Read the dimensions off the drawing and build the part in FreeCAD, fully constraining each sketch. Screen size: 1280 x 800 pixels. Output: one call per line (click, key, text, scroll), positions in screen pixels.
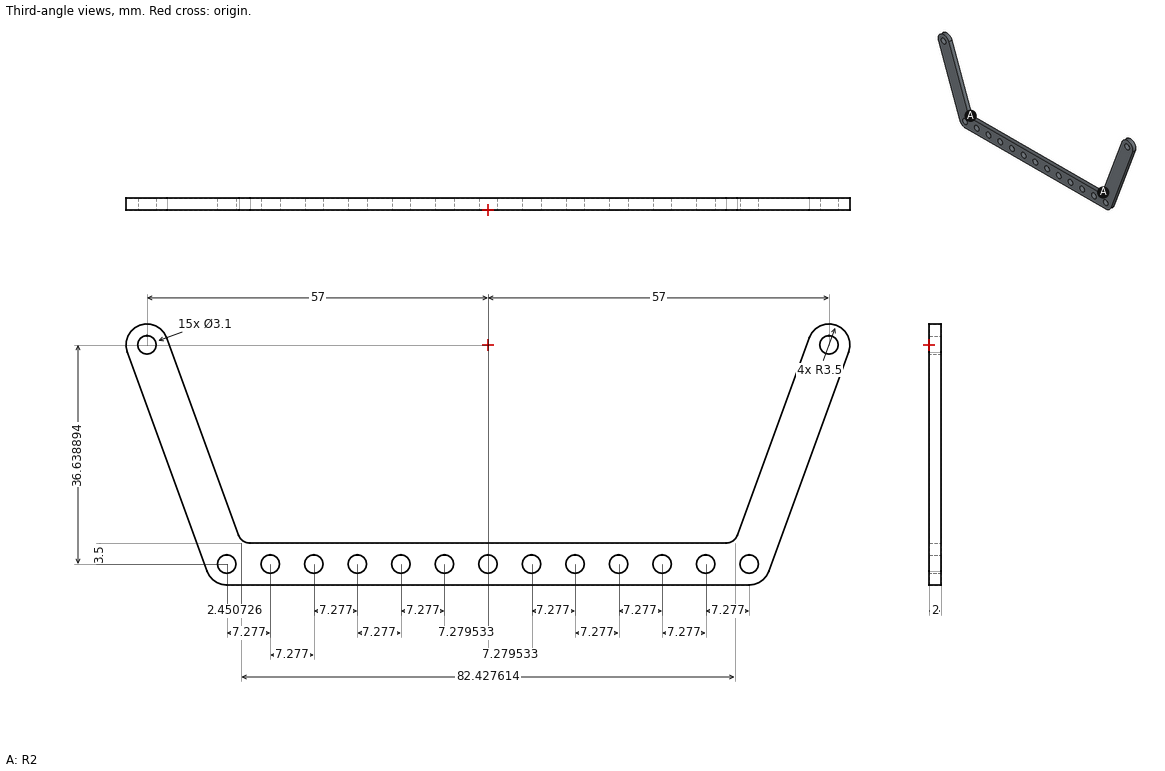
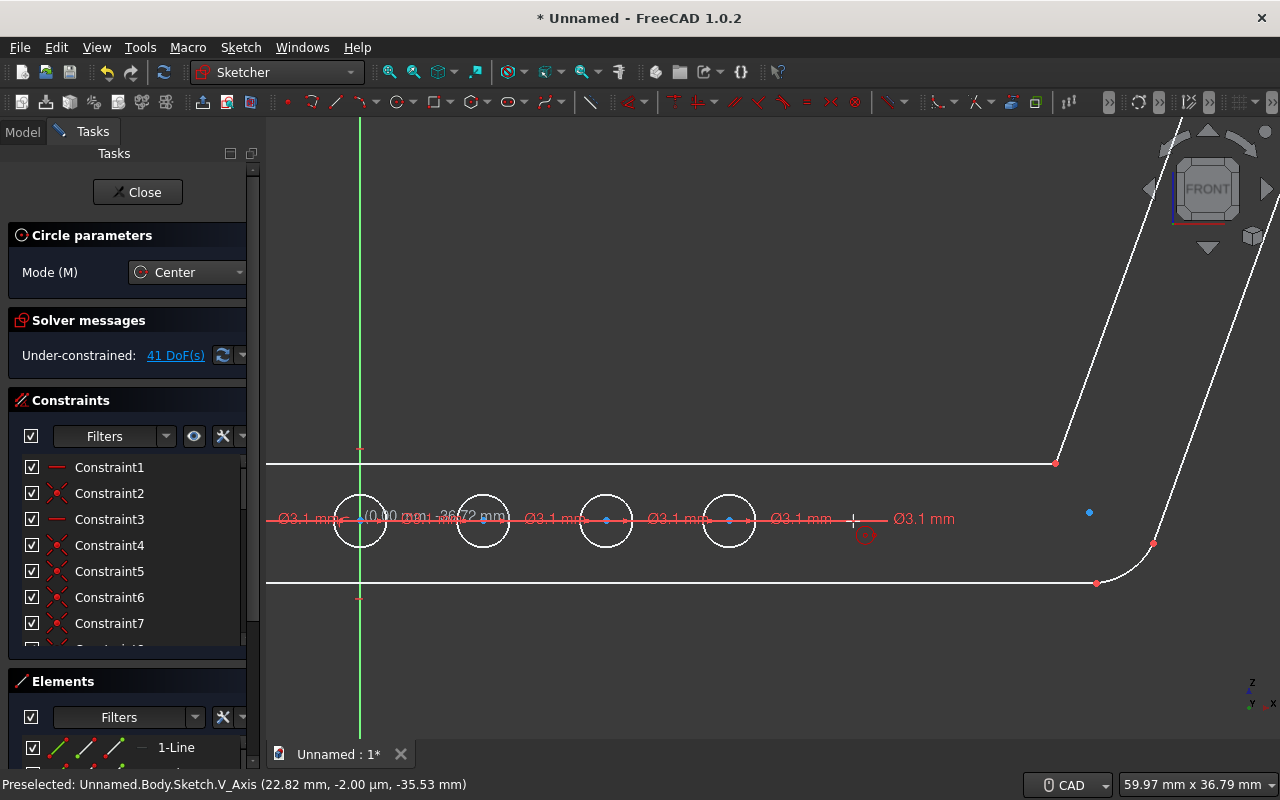
click(852, 520)
move(871, 501)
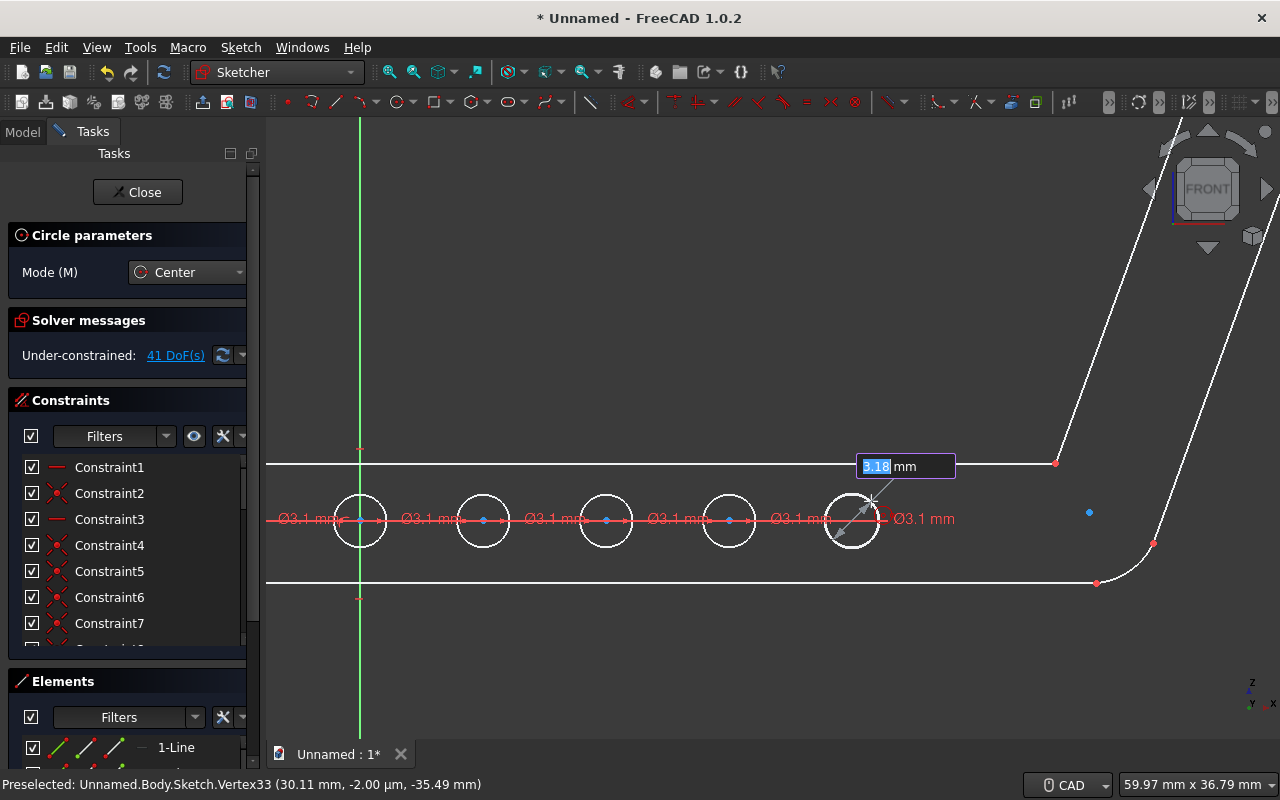
text(3.1)
key(Return)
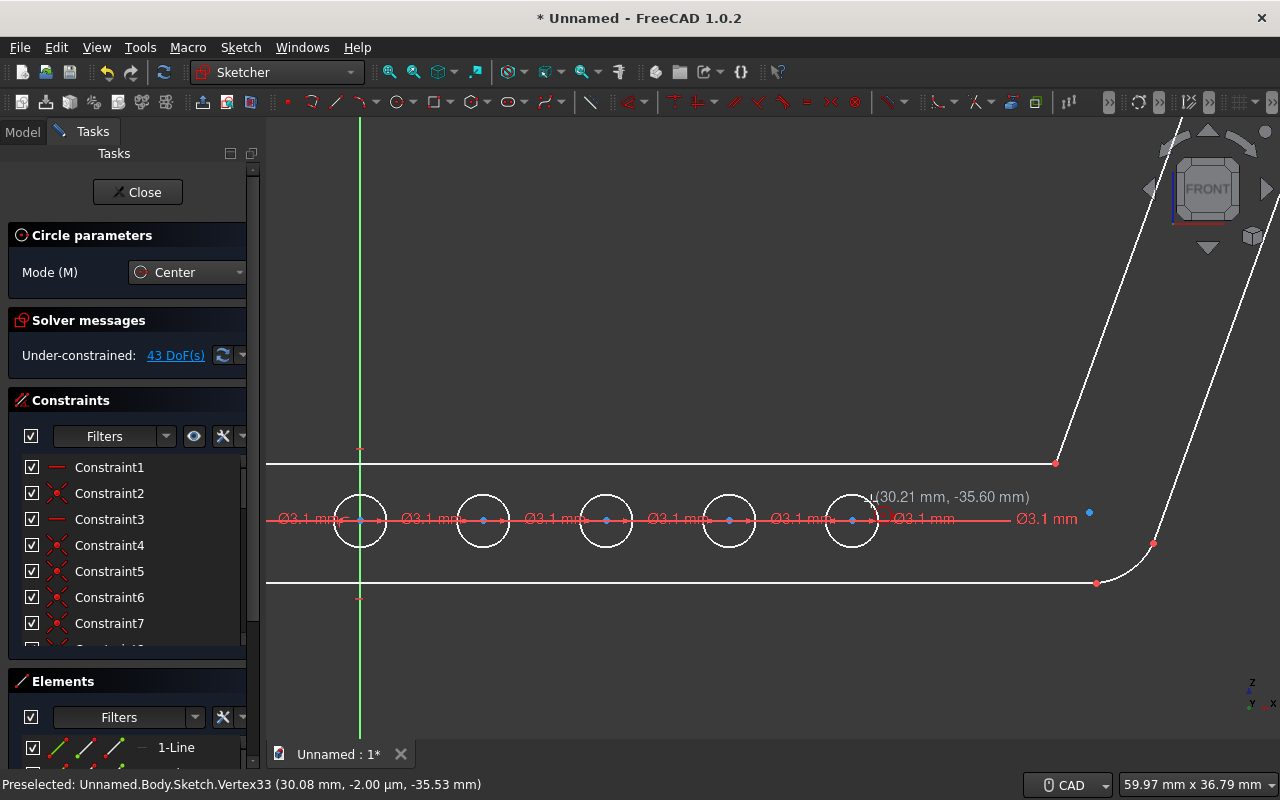
click(975, 520)
move(994, 501)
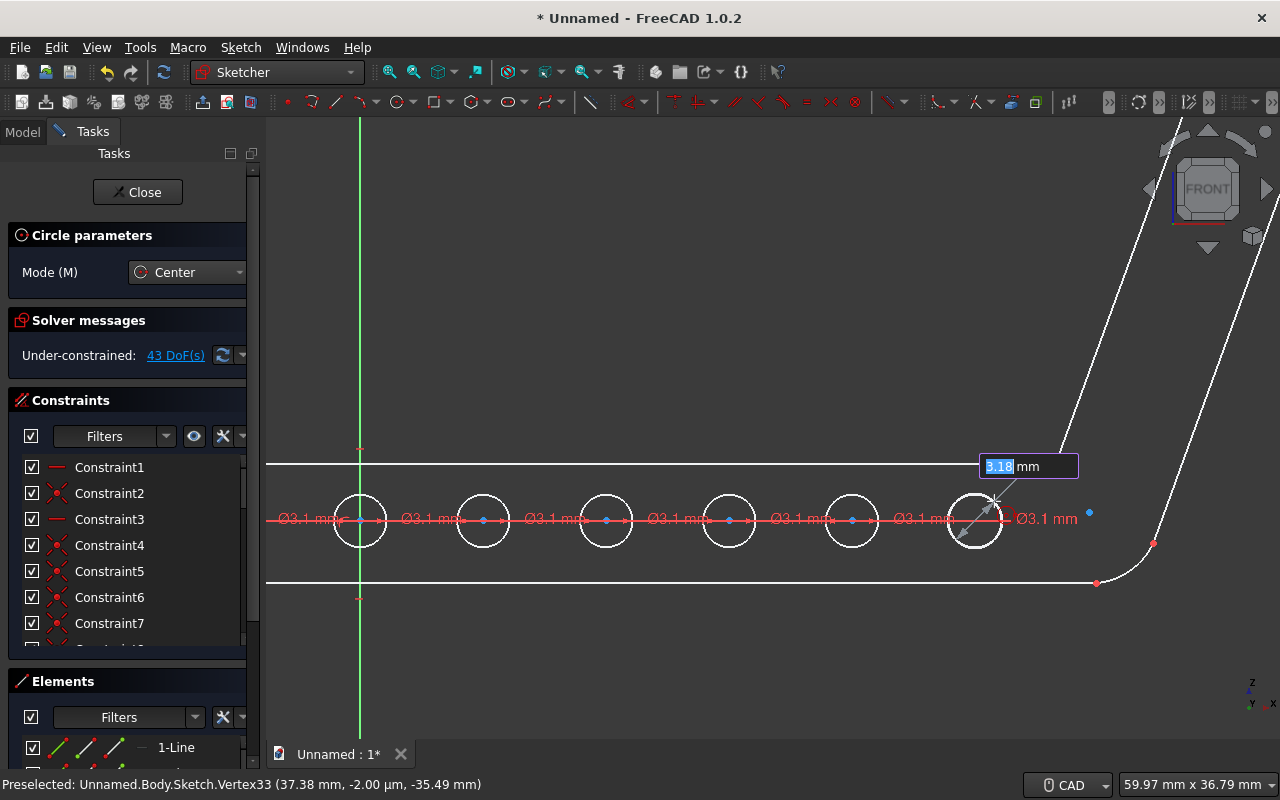
text(3.1)
key(Return)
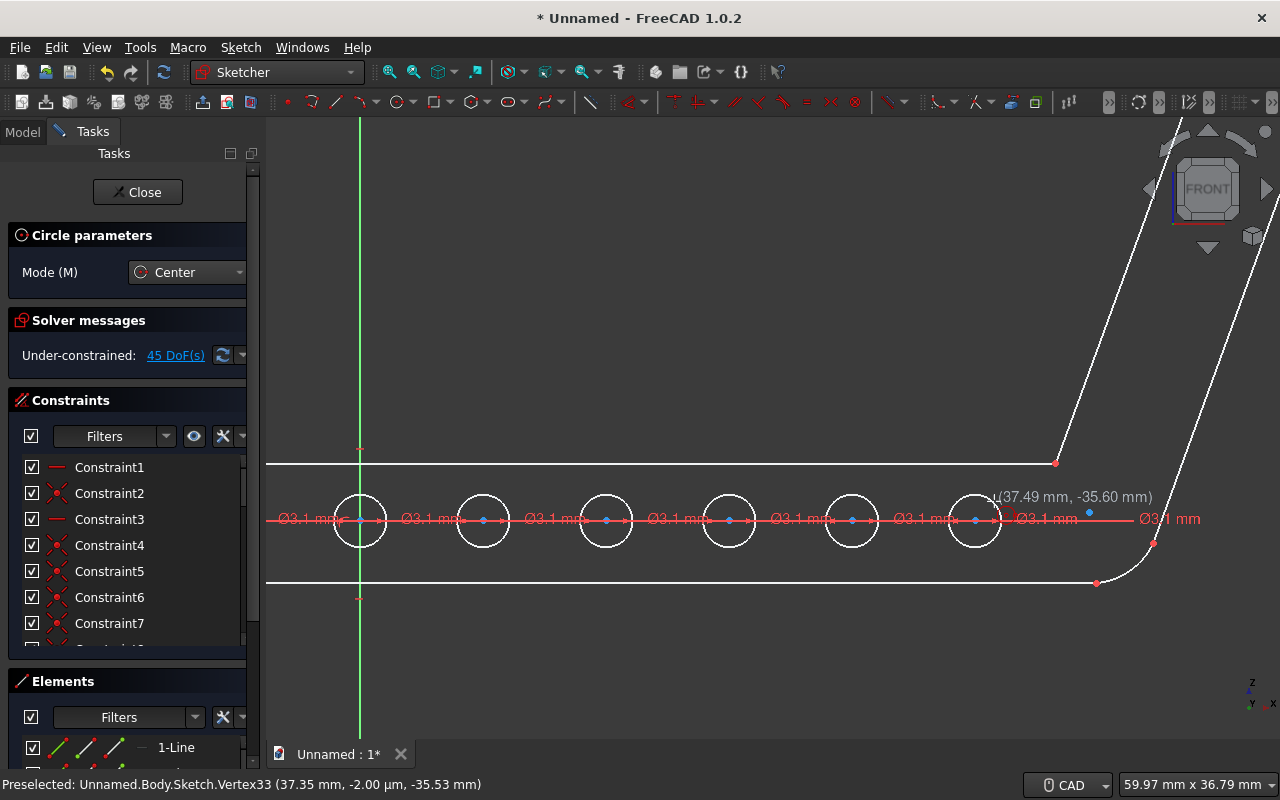
click(1098, 520)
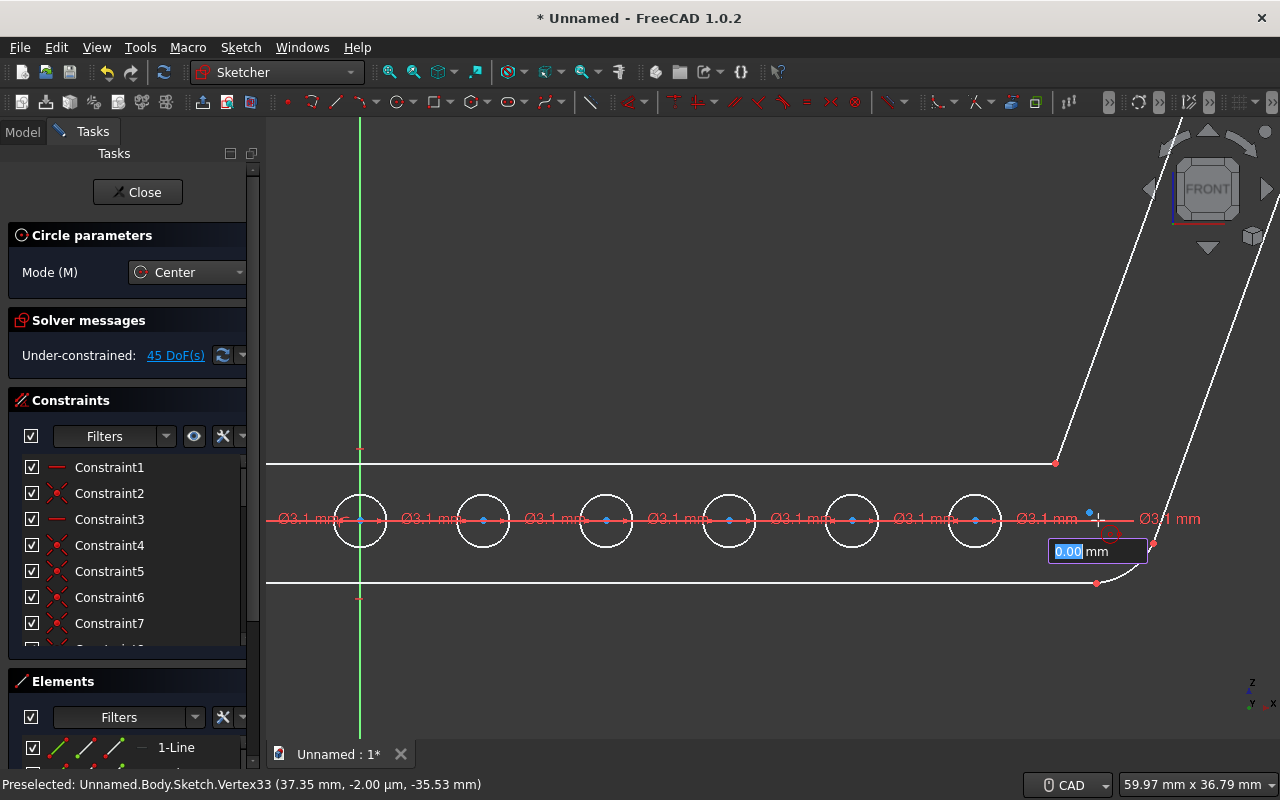
scroll(853, 521, down, 6)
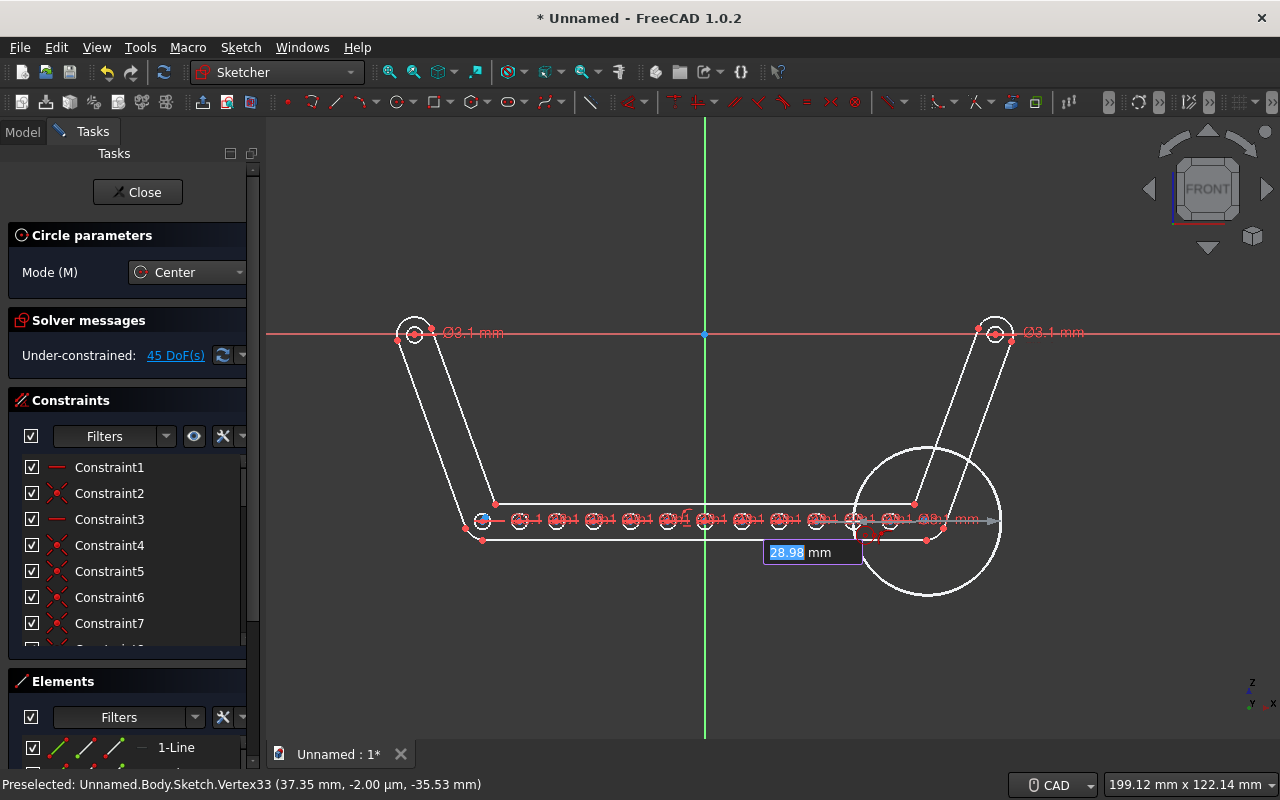
scroll(933, 515, up, 4)
move(932, 515)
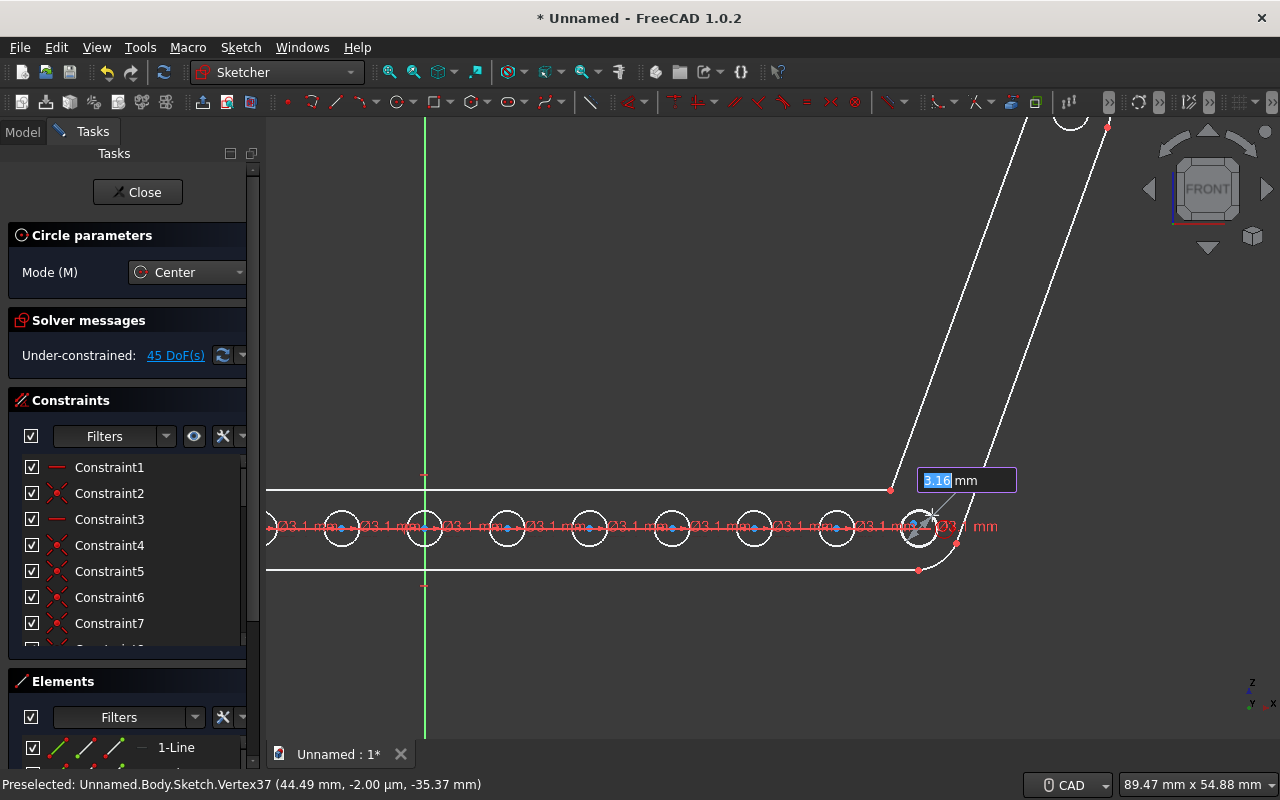
text(3.1)
key(Return)
key(Escape)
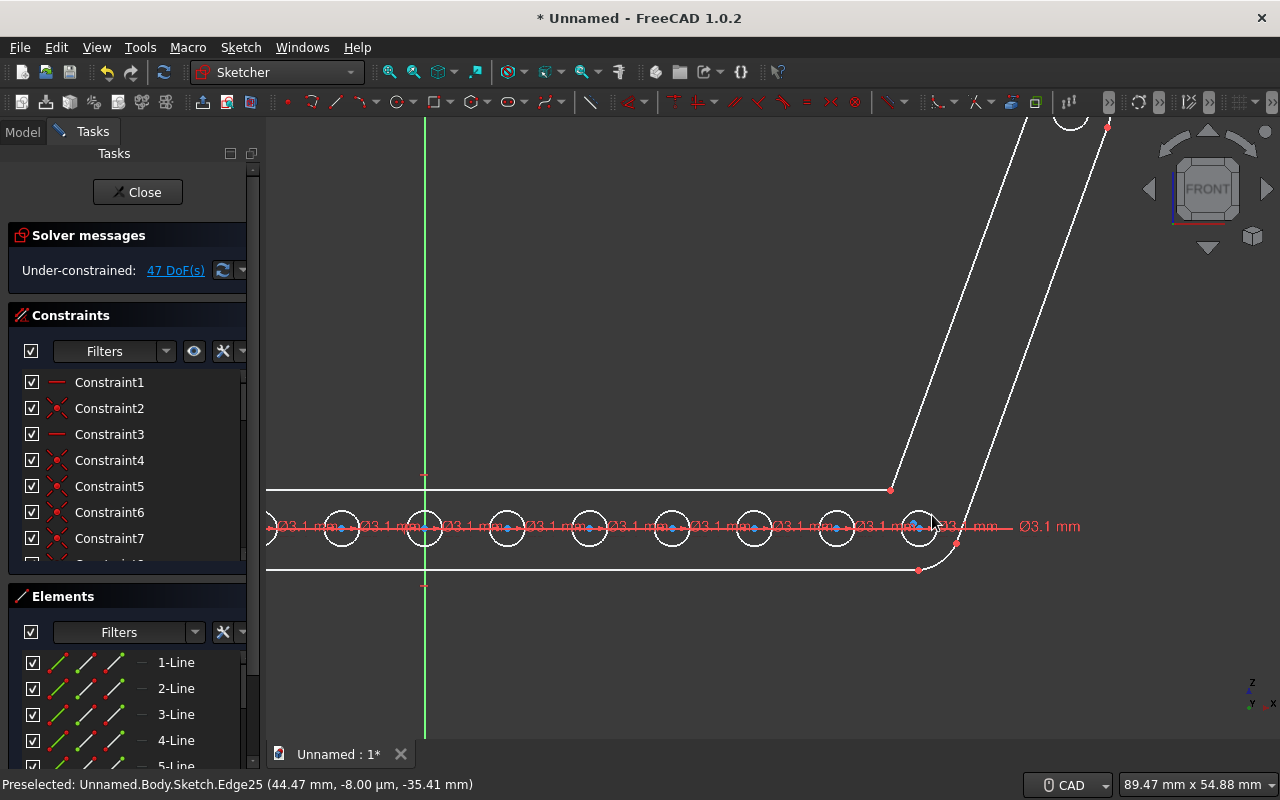
click(1062, 252)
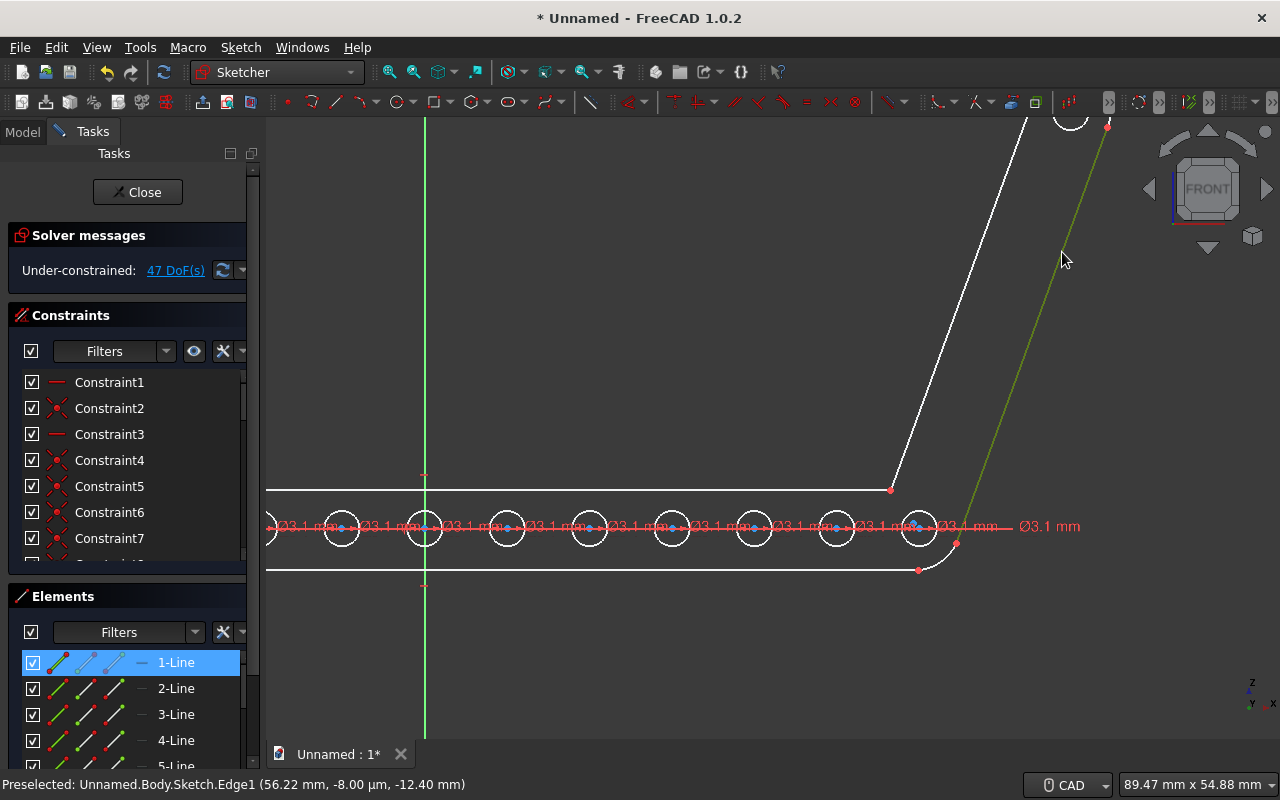
click(932, 567)